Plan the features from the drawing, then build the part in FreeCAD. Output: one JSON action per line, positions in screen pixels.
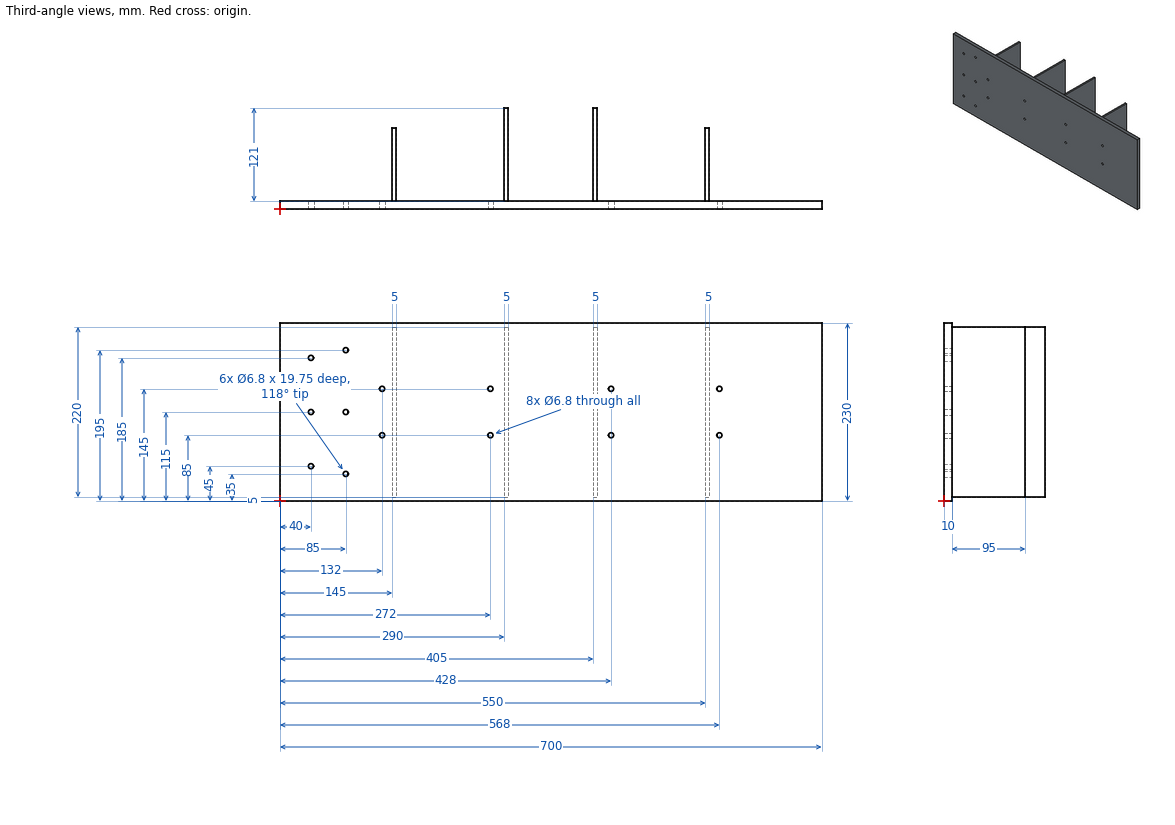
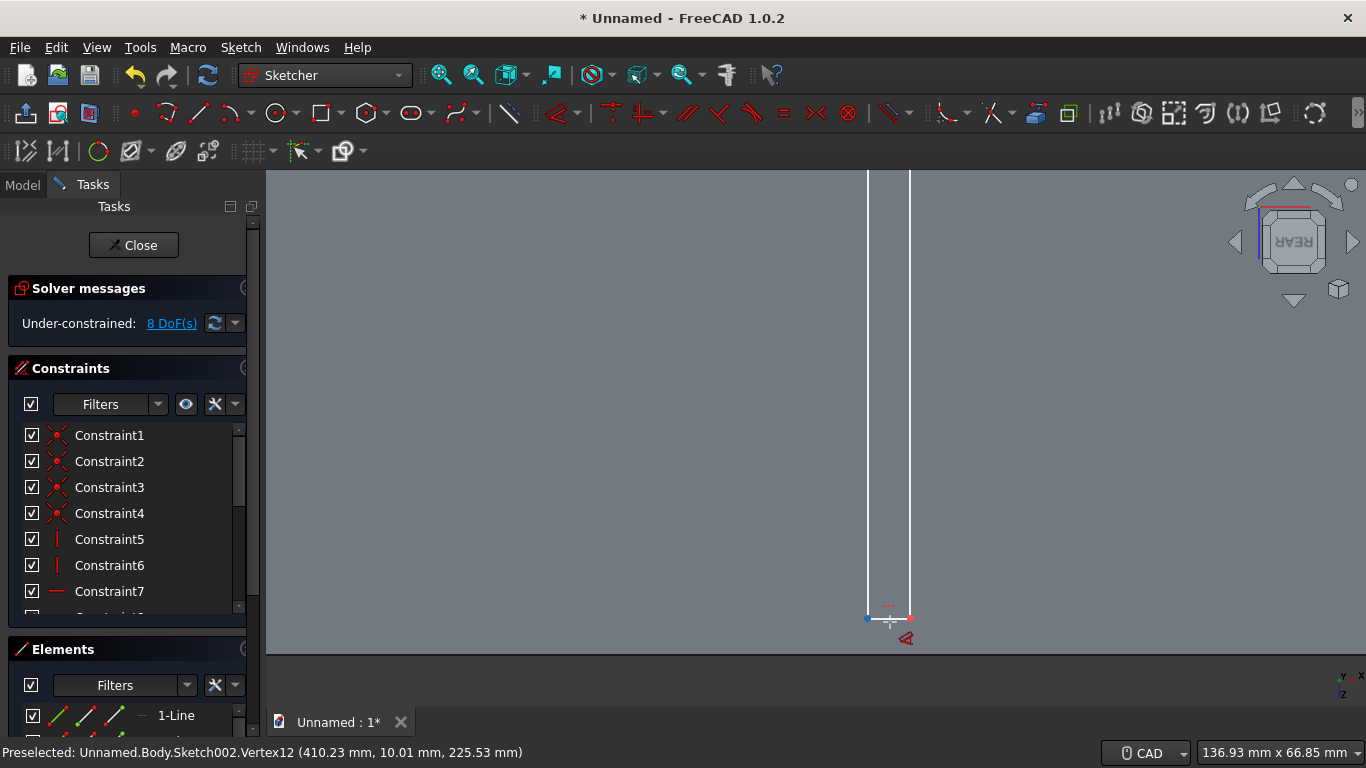
{"action": "left_click", "coordinate": [889, 619]}
{"action": "left_click", "coordinate": [889, 653]}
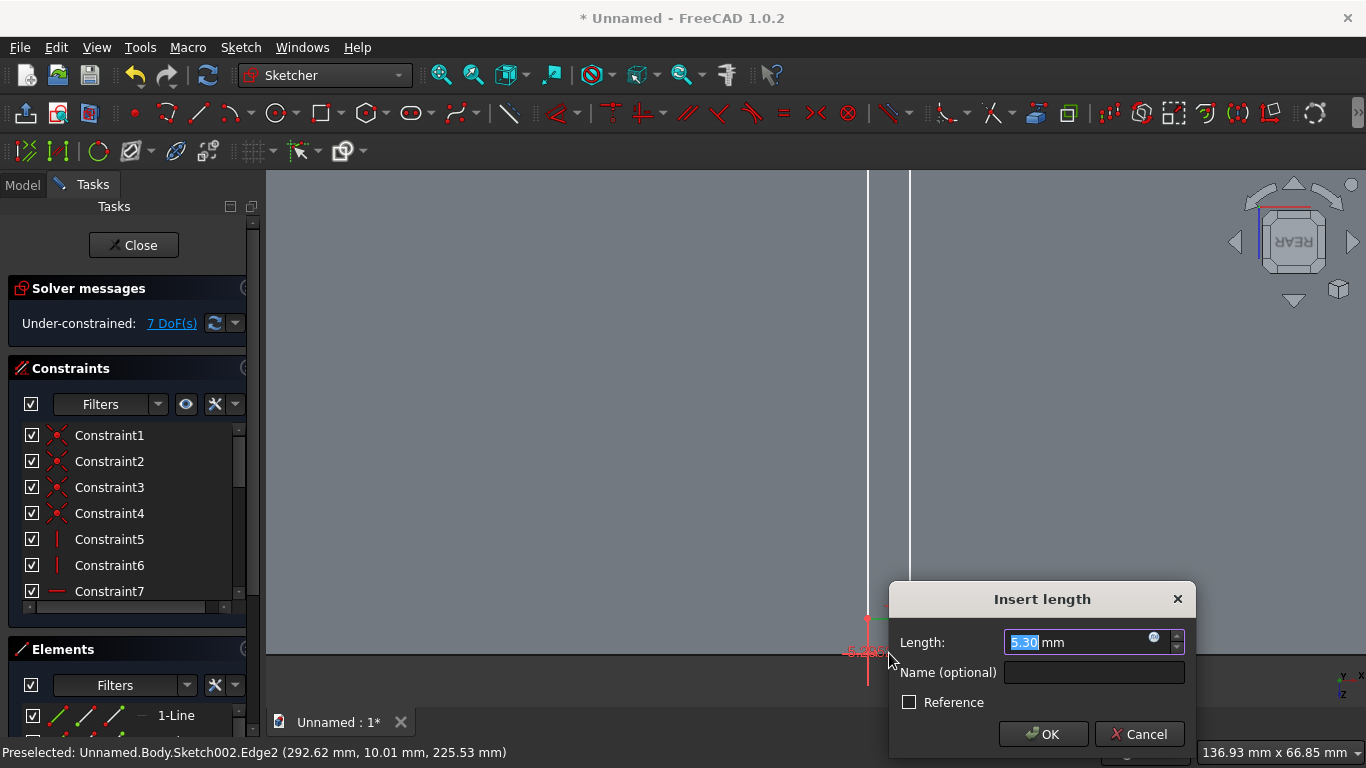
{"action": "type", "text": "5"}
{"action": "key", "text": "Return"}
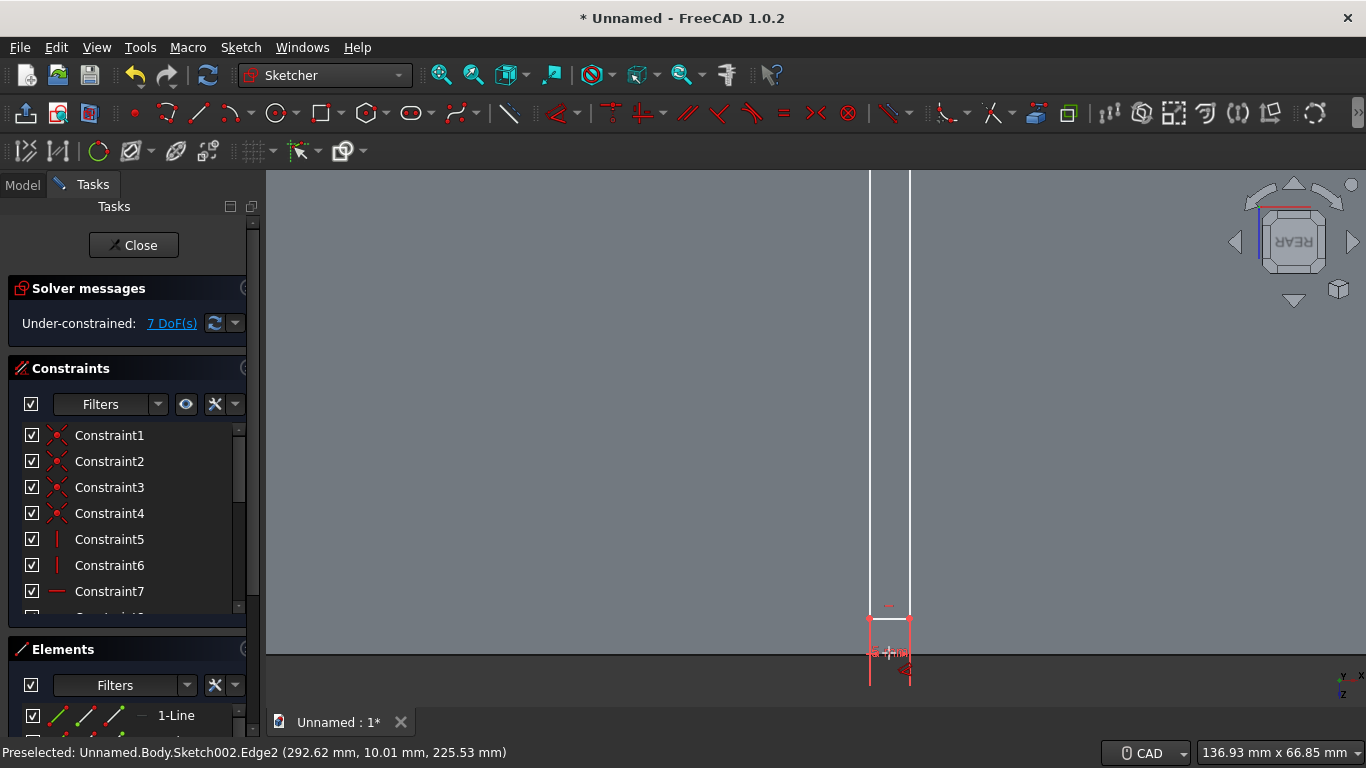
{"action": "scroll", "coordinate": [890, 623], "scroll_direction": "down", "scroll_amount": 8}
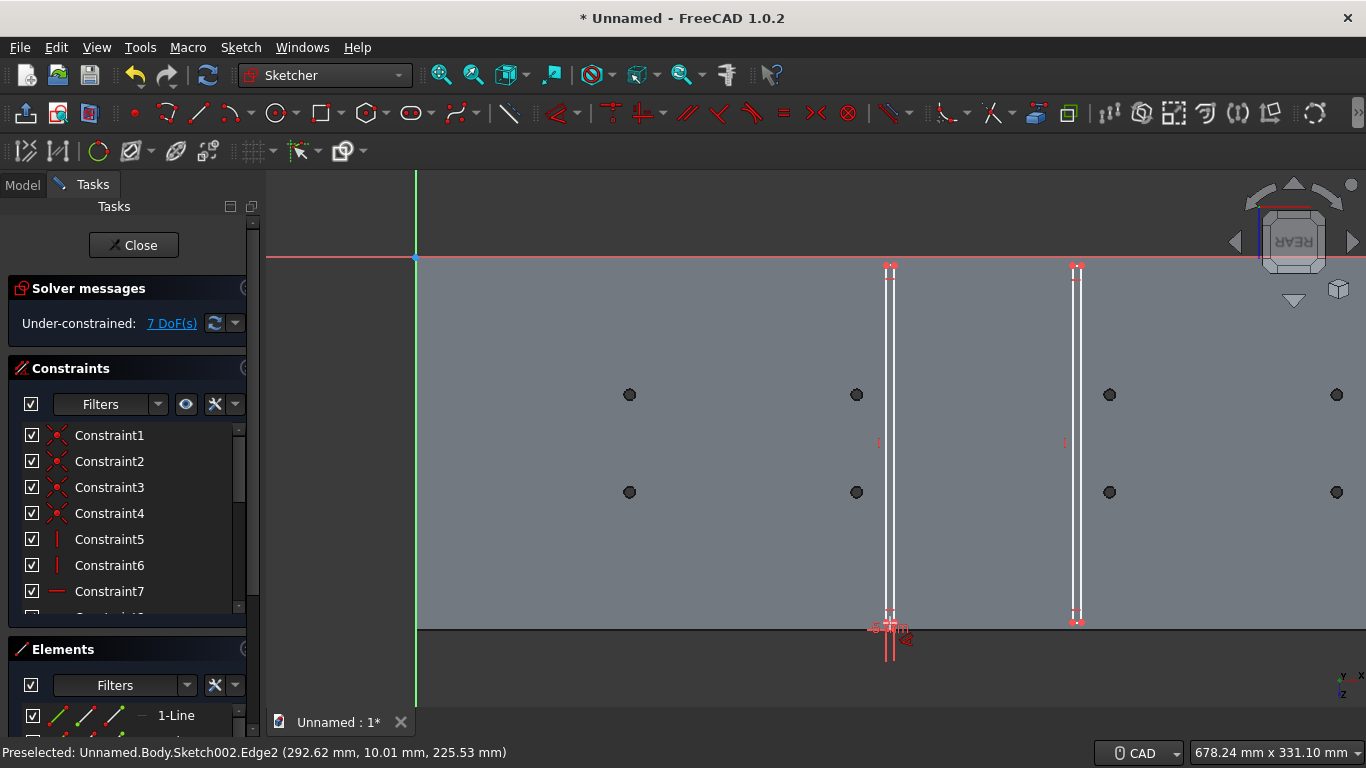
{"action": "scroll", "coordinate": [1075, 623], "scroll_direction": "up", "scroll_amount": 9}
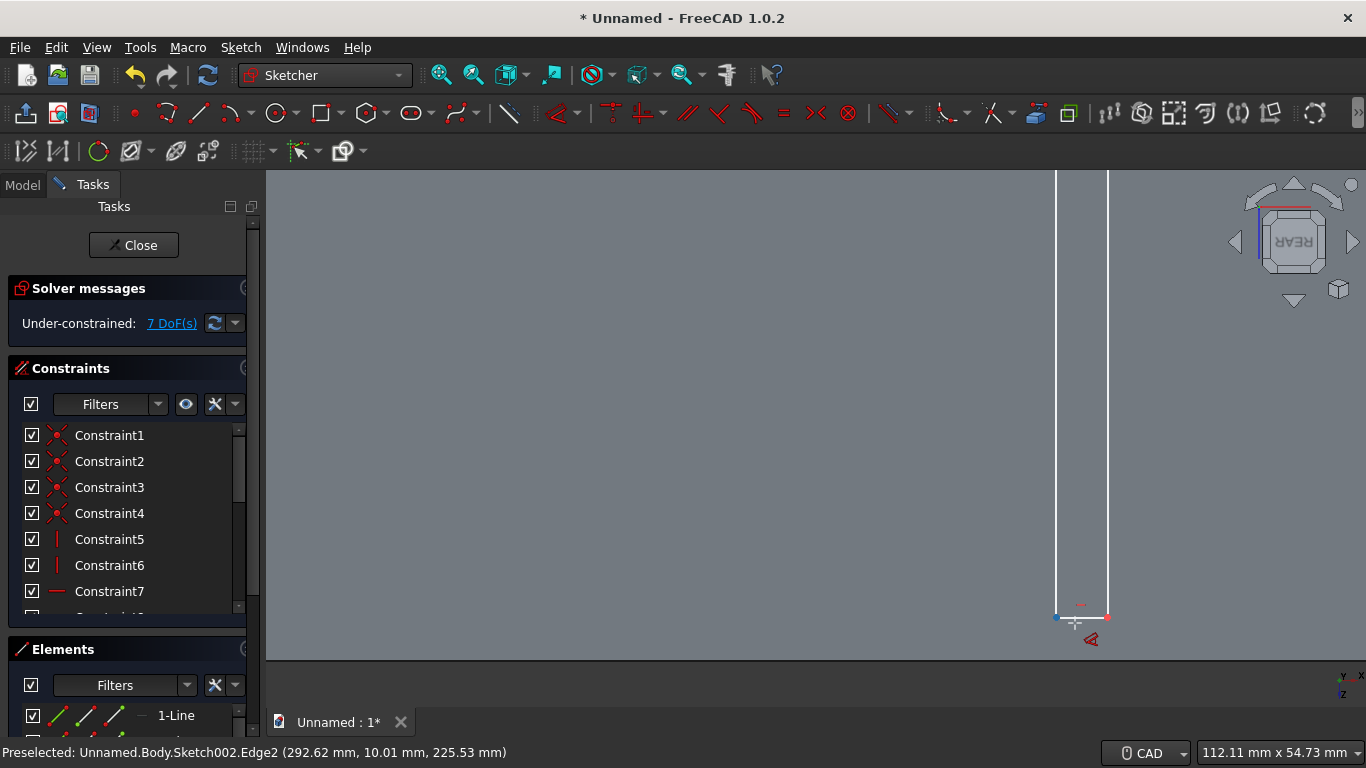
{"action": "left_click", "coordinate": [1072, 618]}
{"action": "left_click", "coordinate": [1082, 652]}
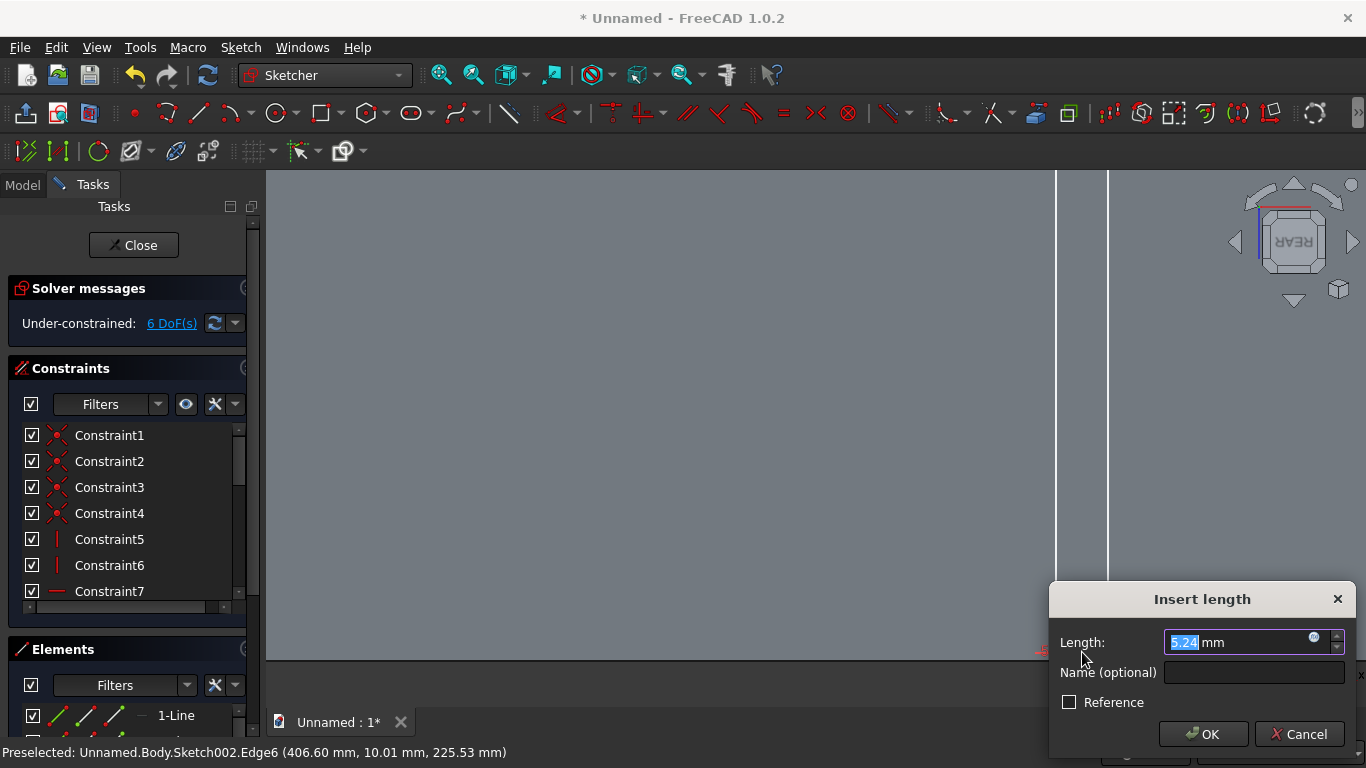
{"action": "type", "text": "5"}
{"action": "key", "text": "Return"}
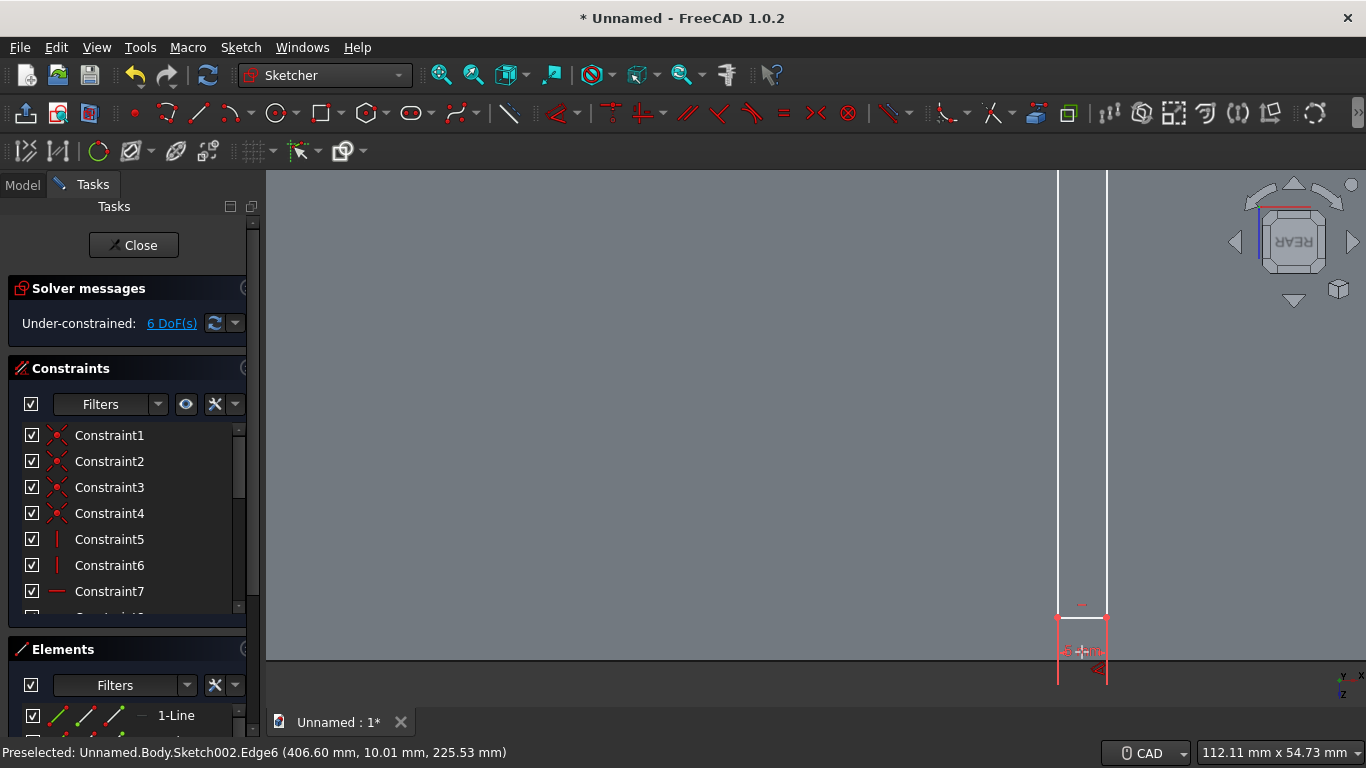
{"action": "scroll", "coordinate": [1075, 623], "scroll_direction": "down", "scroll_amount": 9}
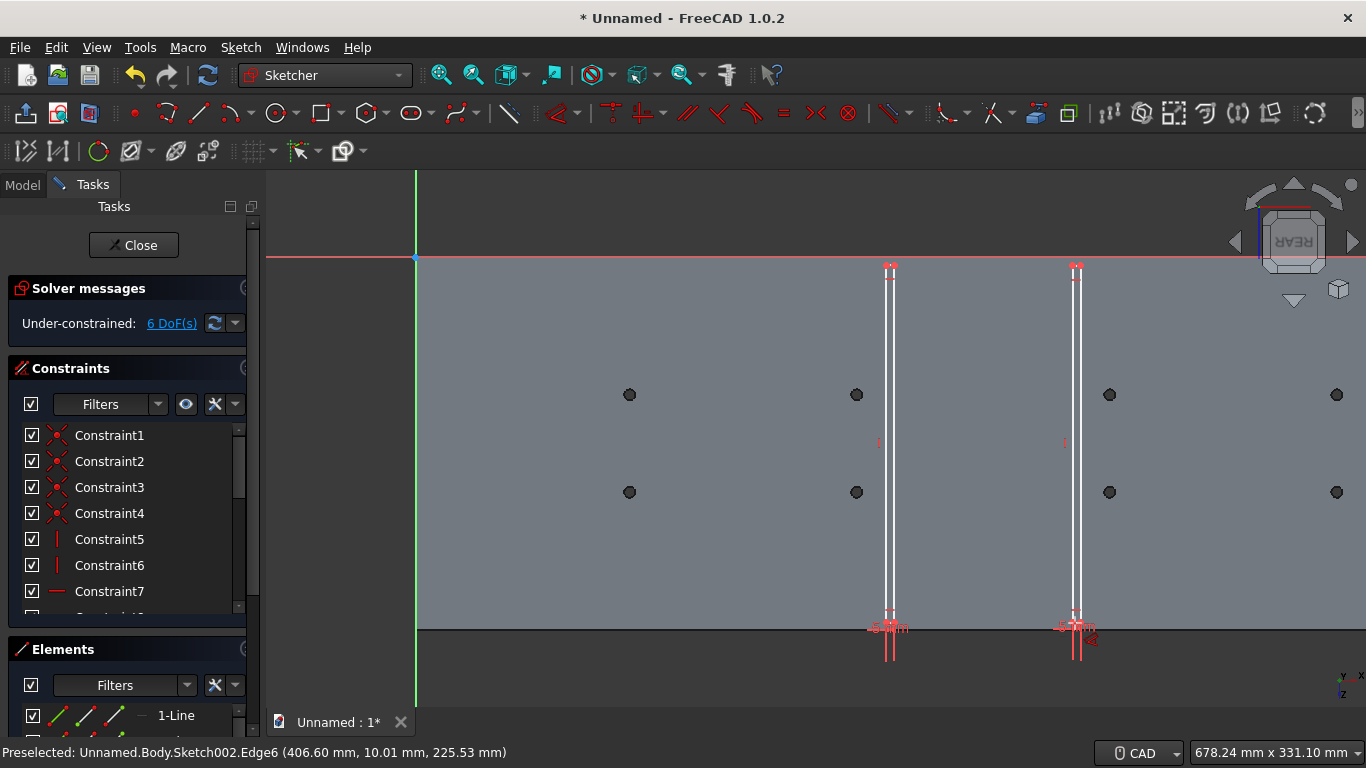
{"action": "scroll", "coordinate": [886, 265], "scroll_direction": "up", "scroll_amount": 8}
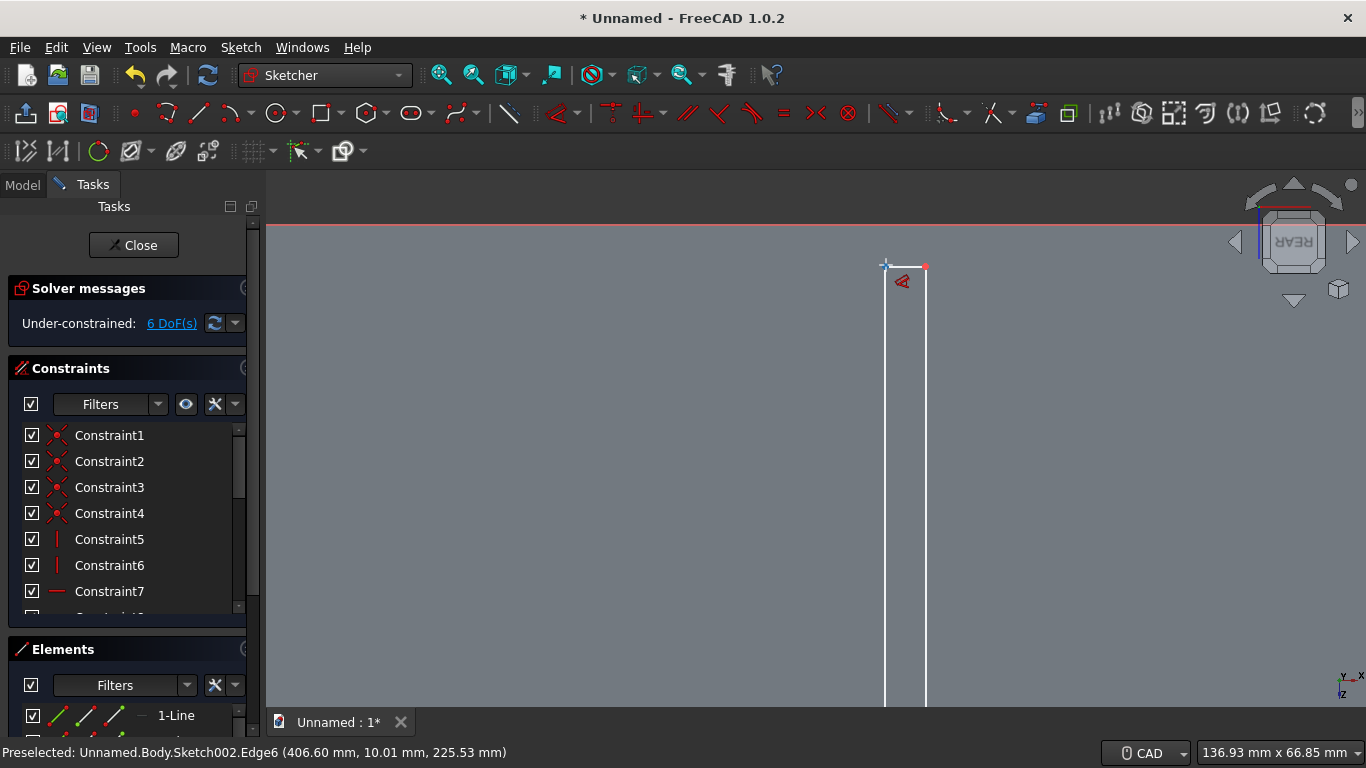
{"action": "left_click", "coordinate": [885, 267]}
{"action": "left_click", "coordinate": [919, 246]}